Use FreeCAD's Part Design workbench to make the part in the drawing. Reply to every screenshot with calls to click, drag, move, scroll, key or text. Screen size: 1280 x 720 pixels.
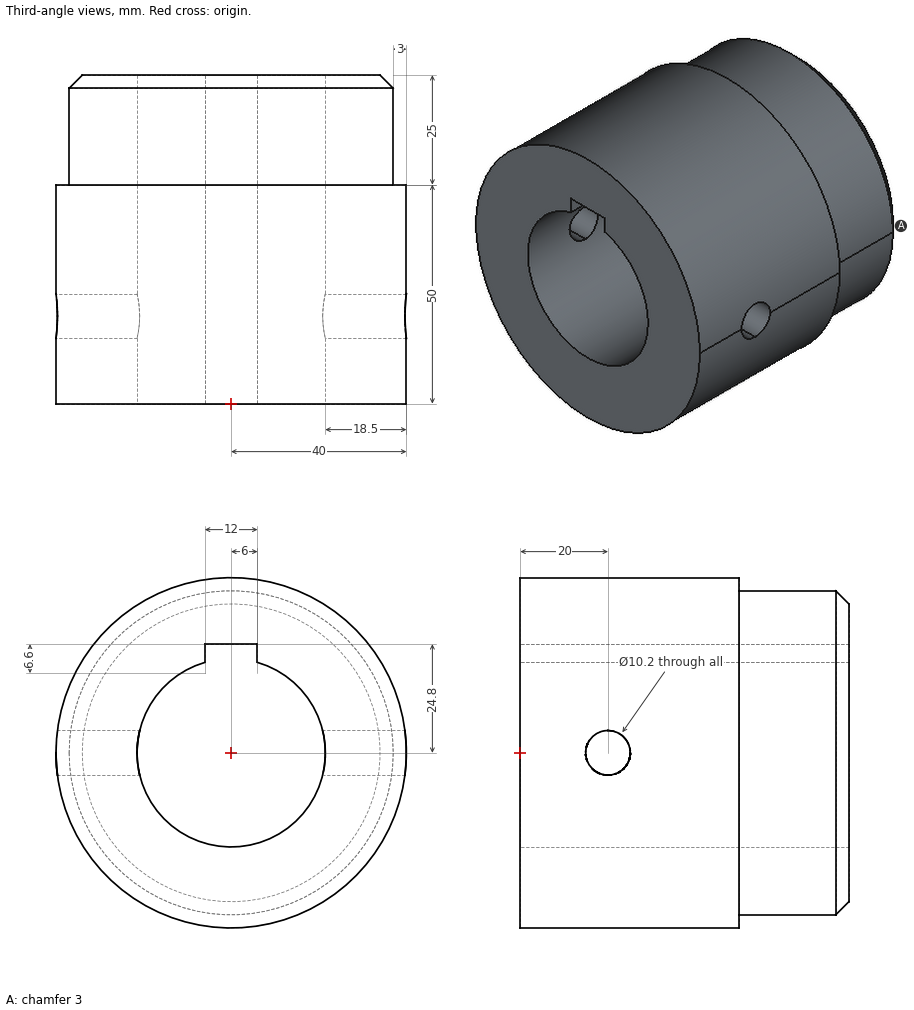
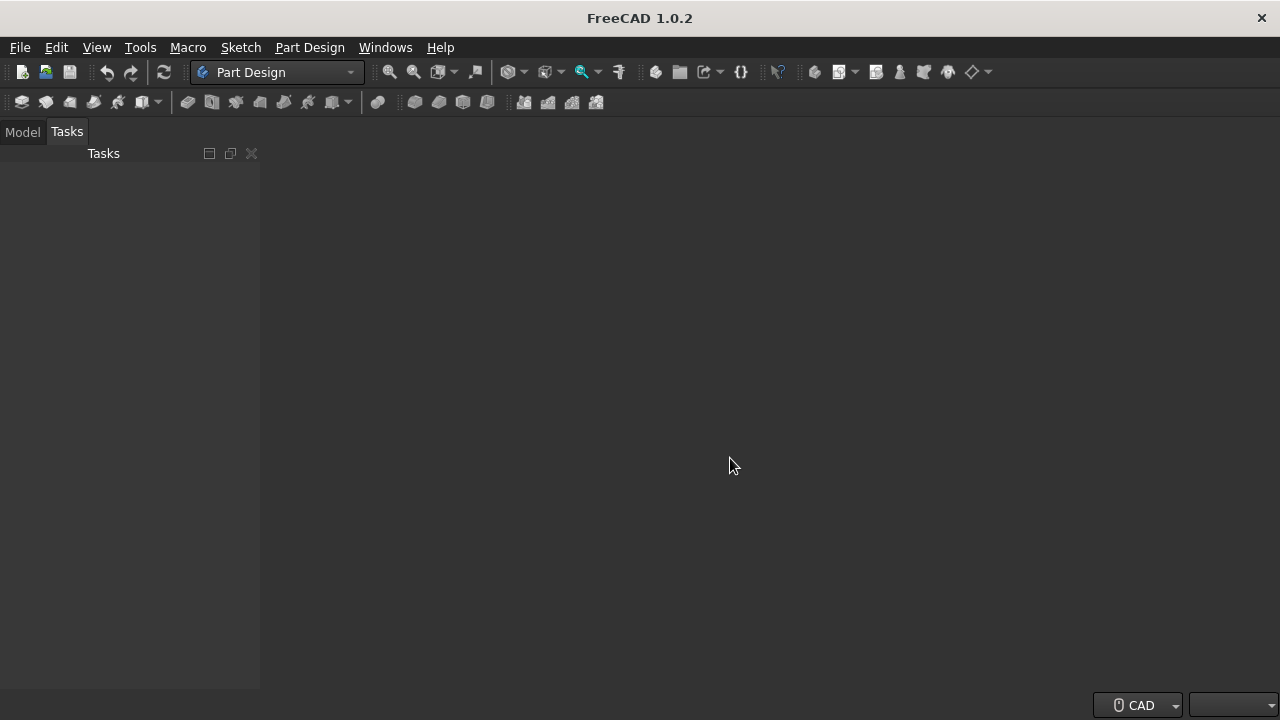
click(22, 72)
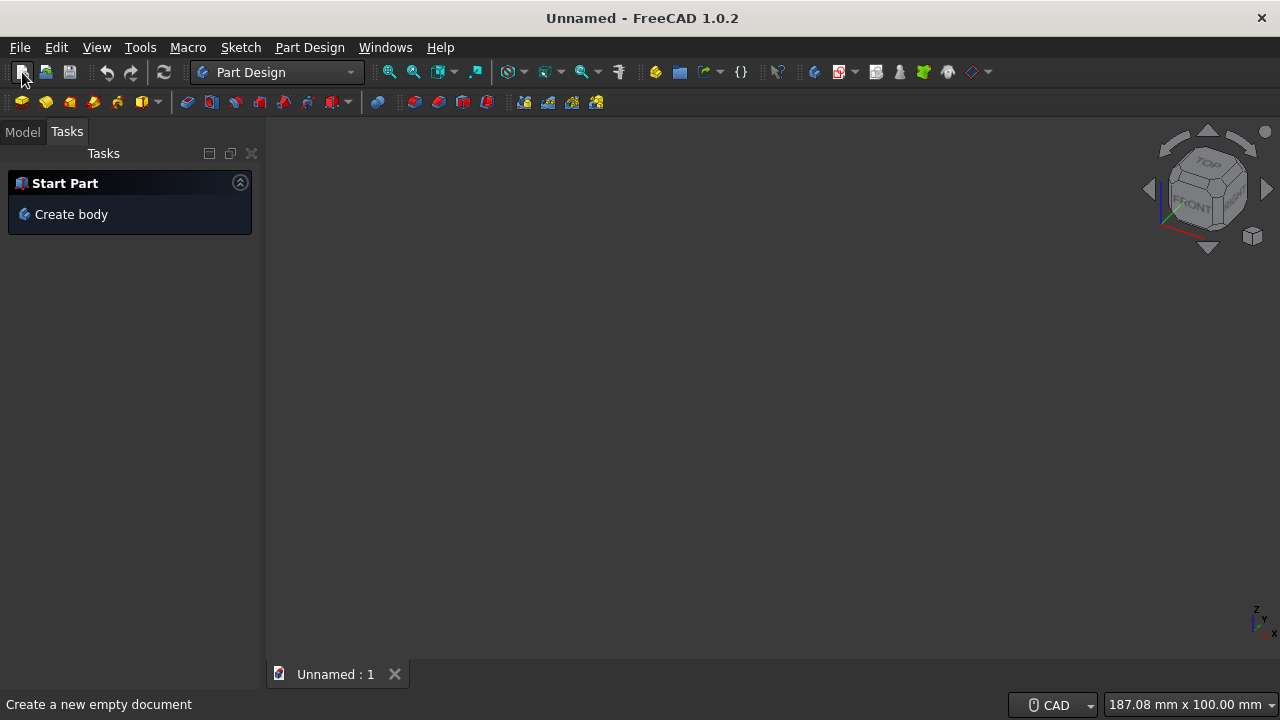
click(840, 72)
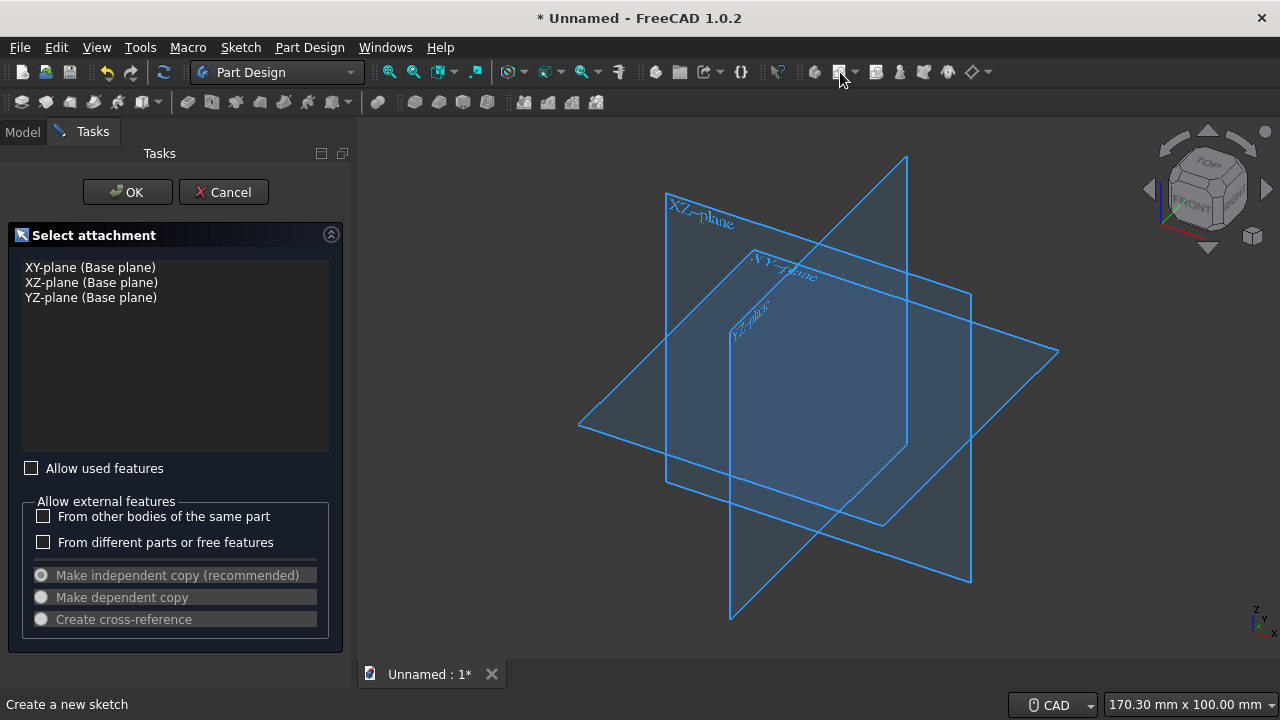
click(82, 268)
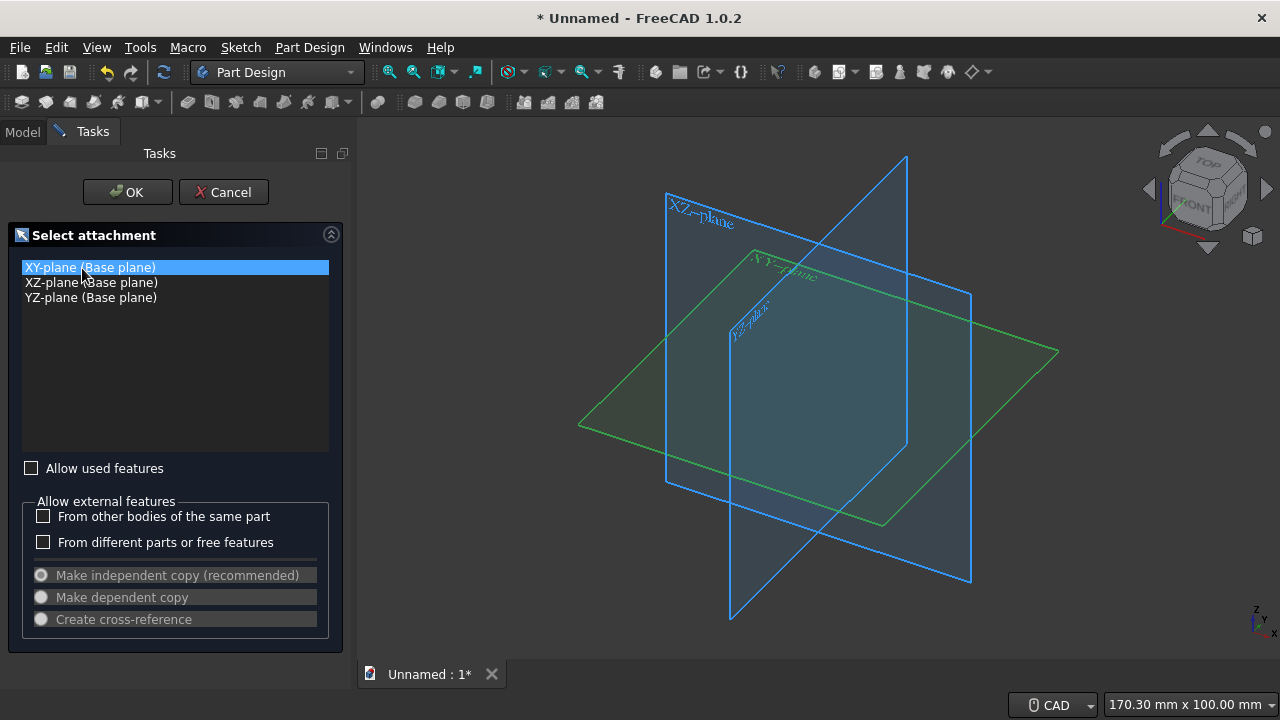
click(128, 192)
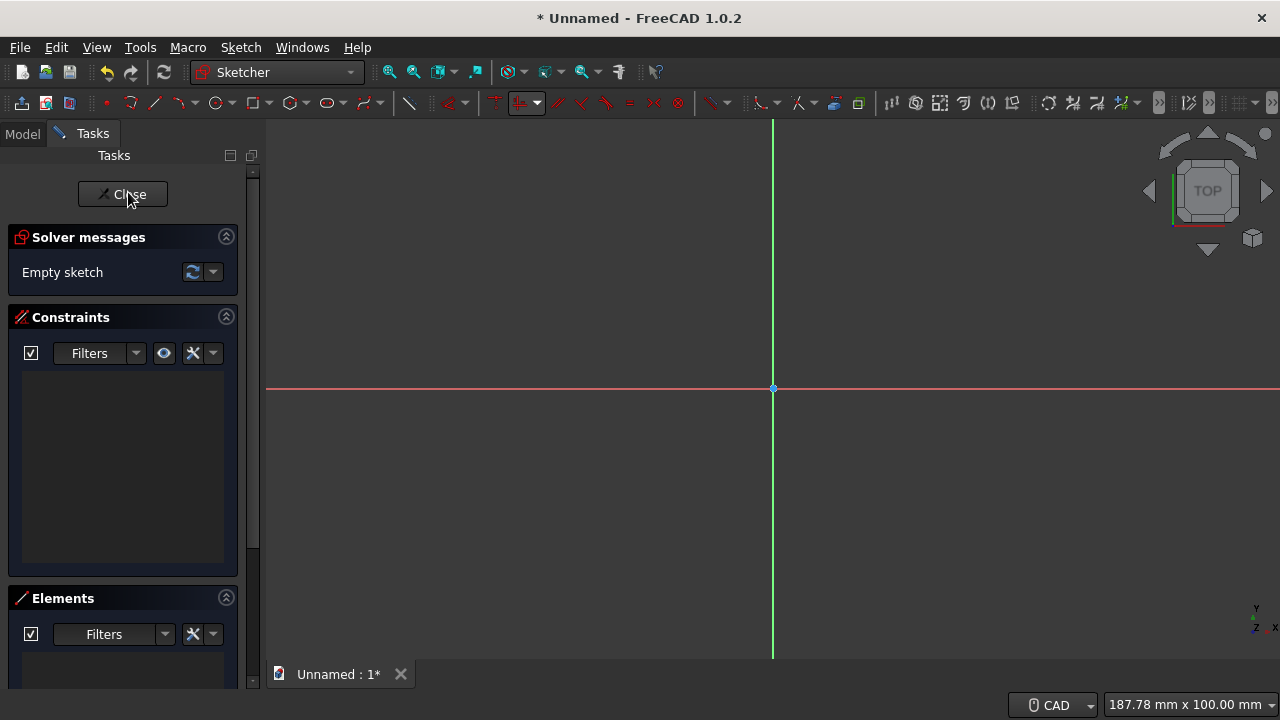
scroll(346, 631, down, 2)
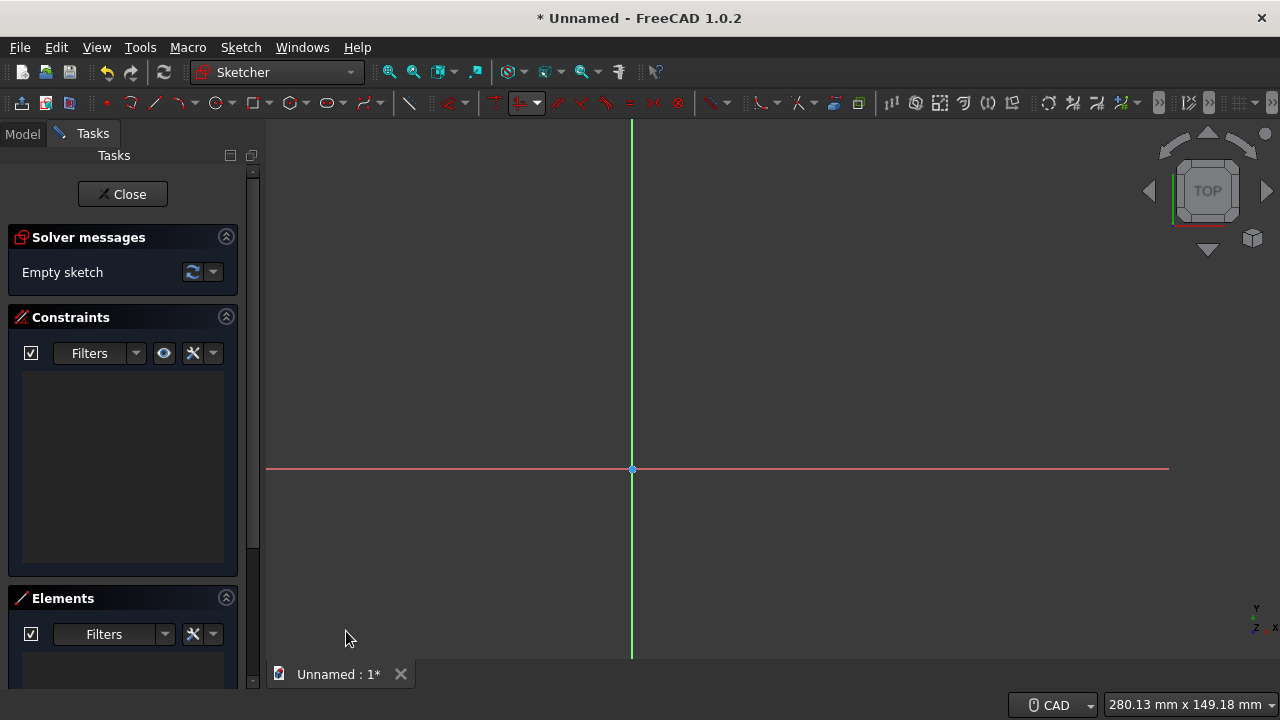
click(132, 104)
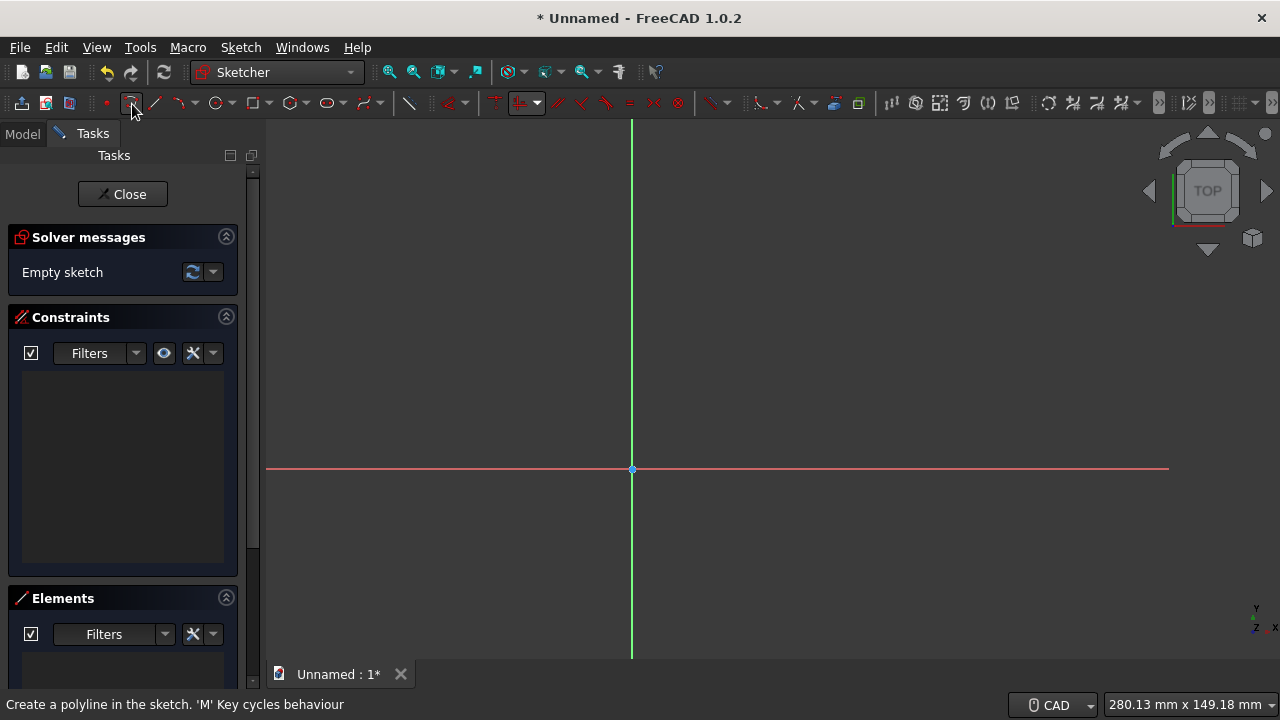
click(710, 469)
click(777, 460)
click(777, 288)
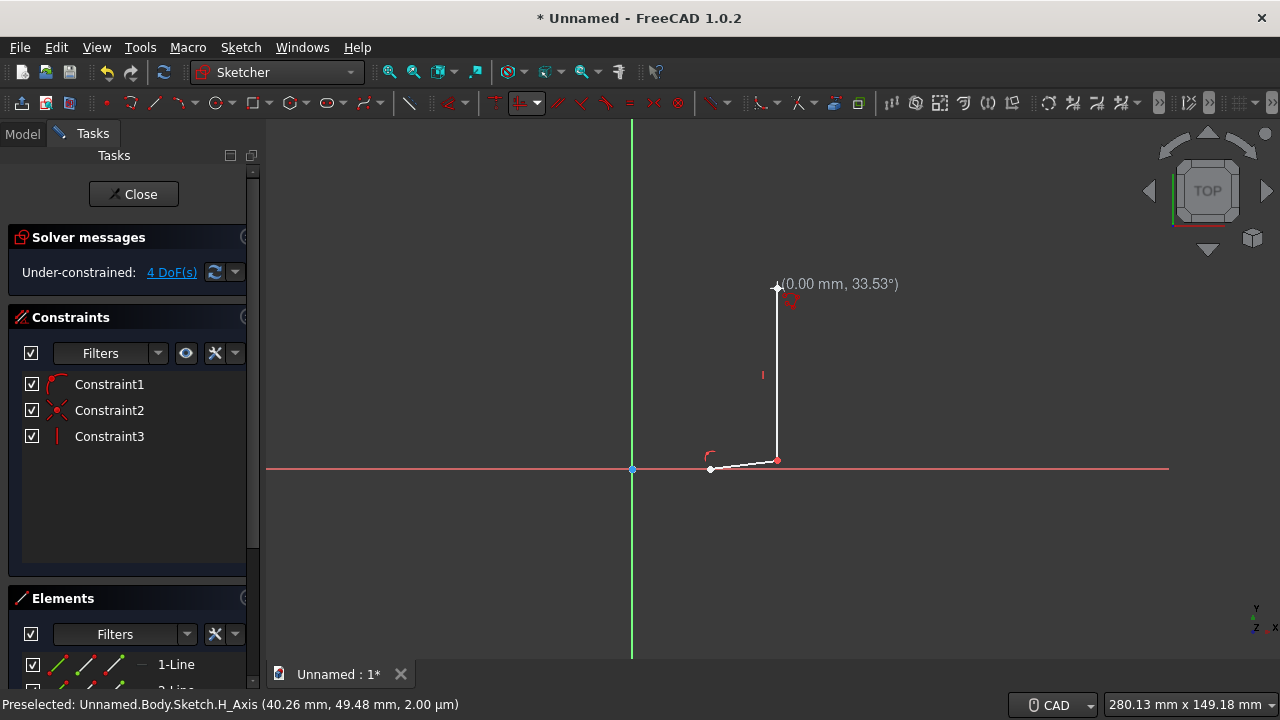
scroll(766, 288, up, 2)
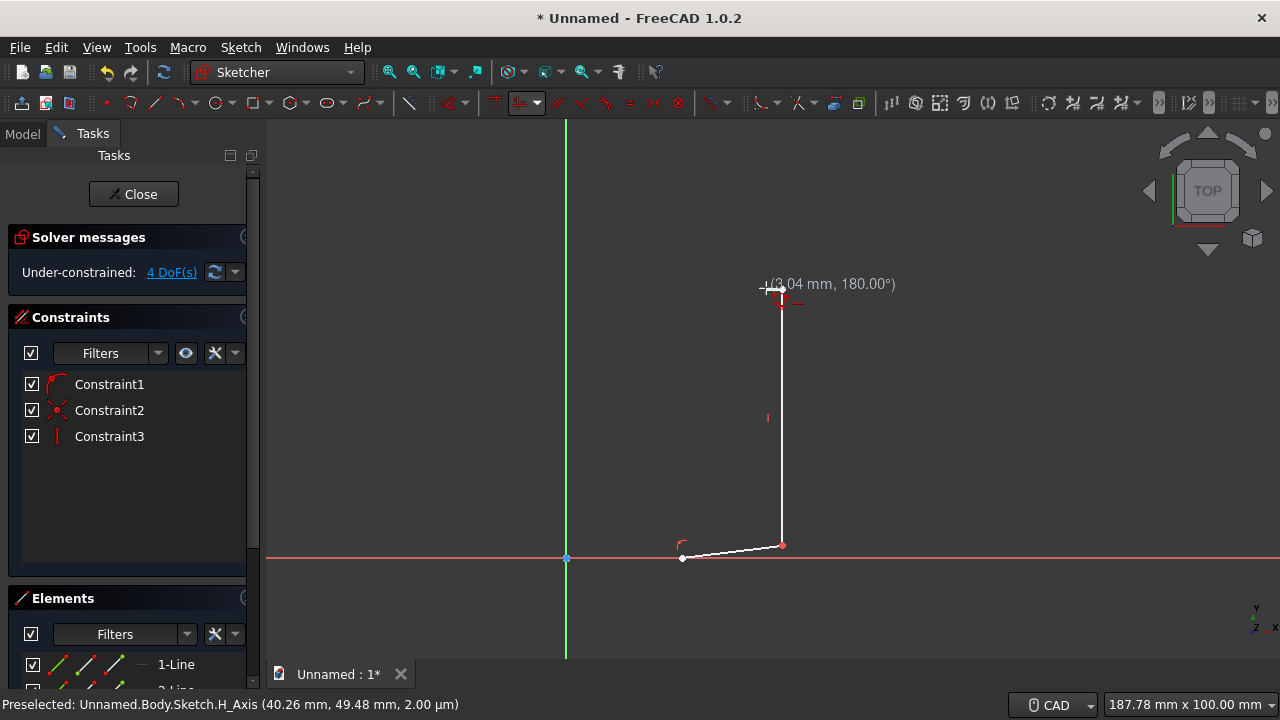
click(766, 288)
click(766, 153)
click(682, 153)
click(682, 558)
key(Escape)
key(Escape)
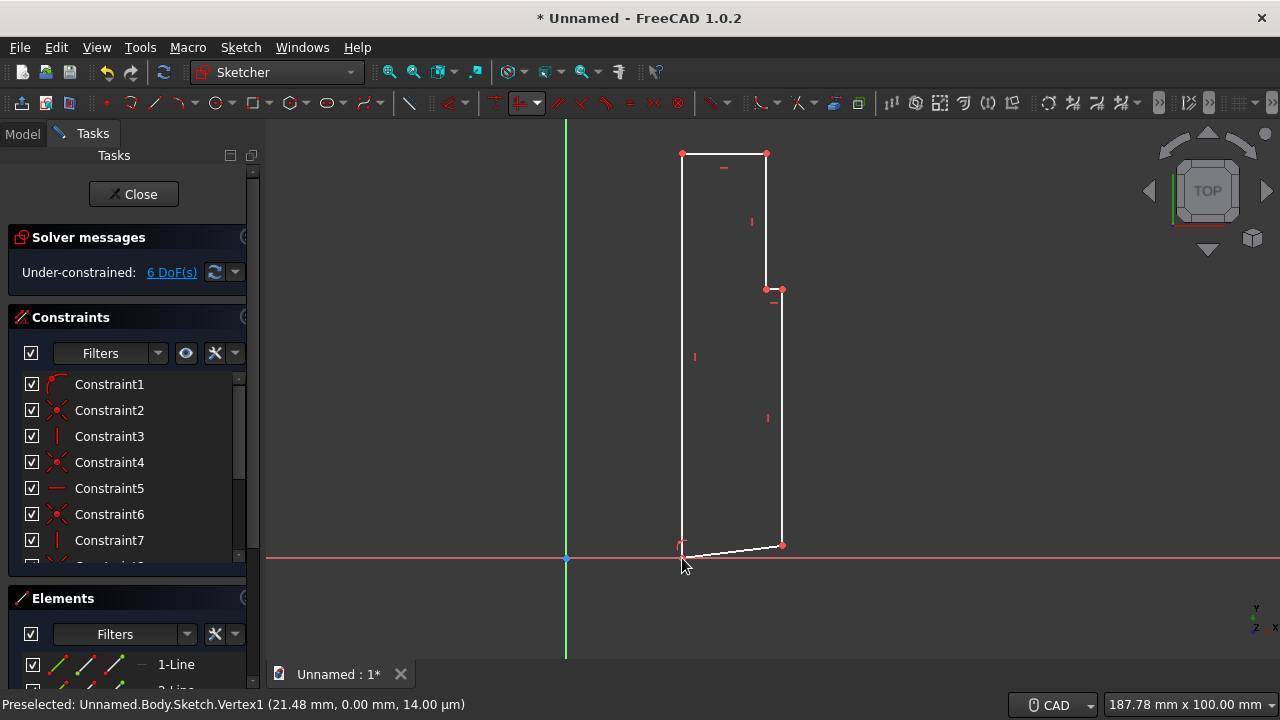
click(712, 554)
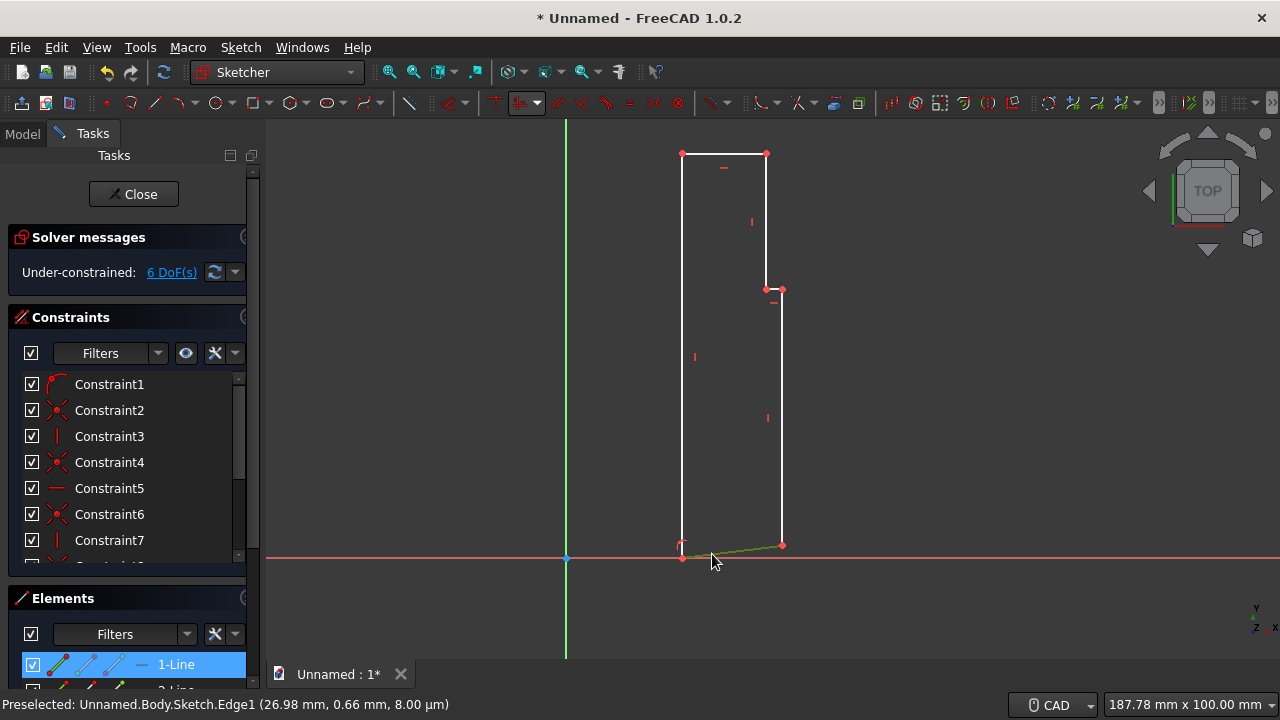
click(540, 104)